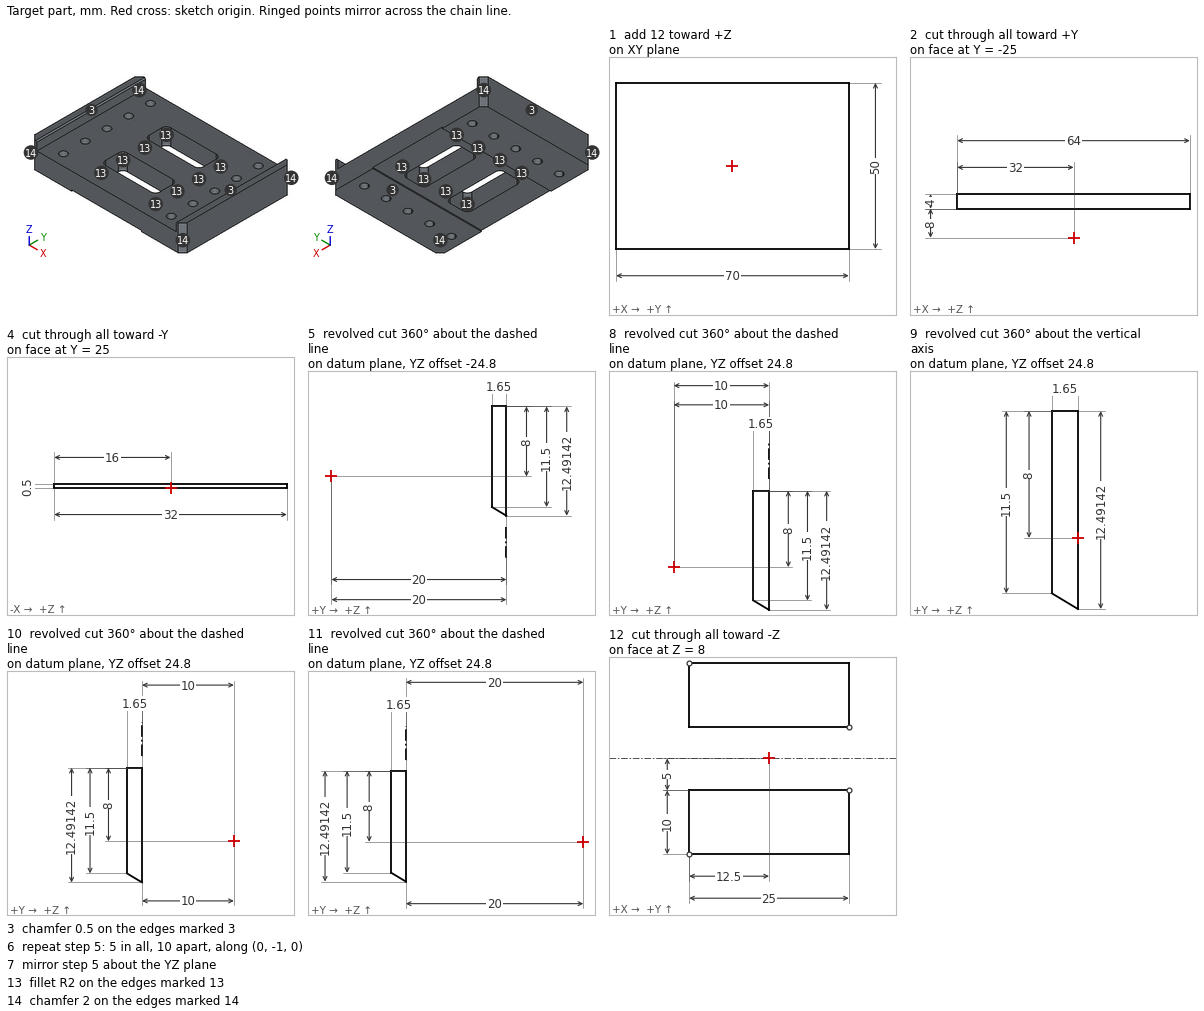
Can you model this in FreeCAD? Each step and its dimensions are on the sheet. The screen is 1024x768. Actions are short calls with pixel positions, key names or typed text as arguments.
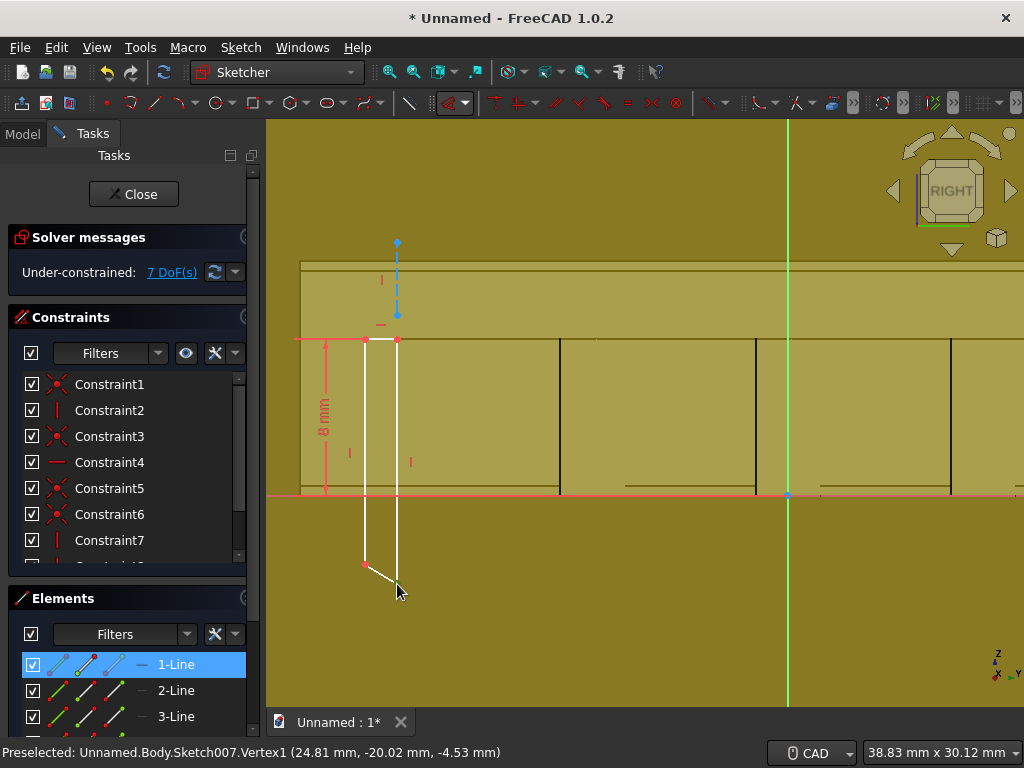
key(l)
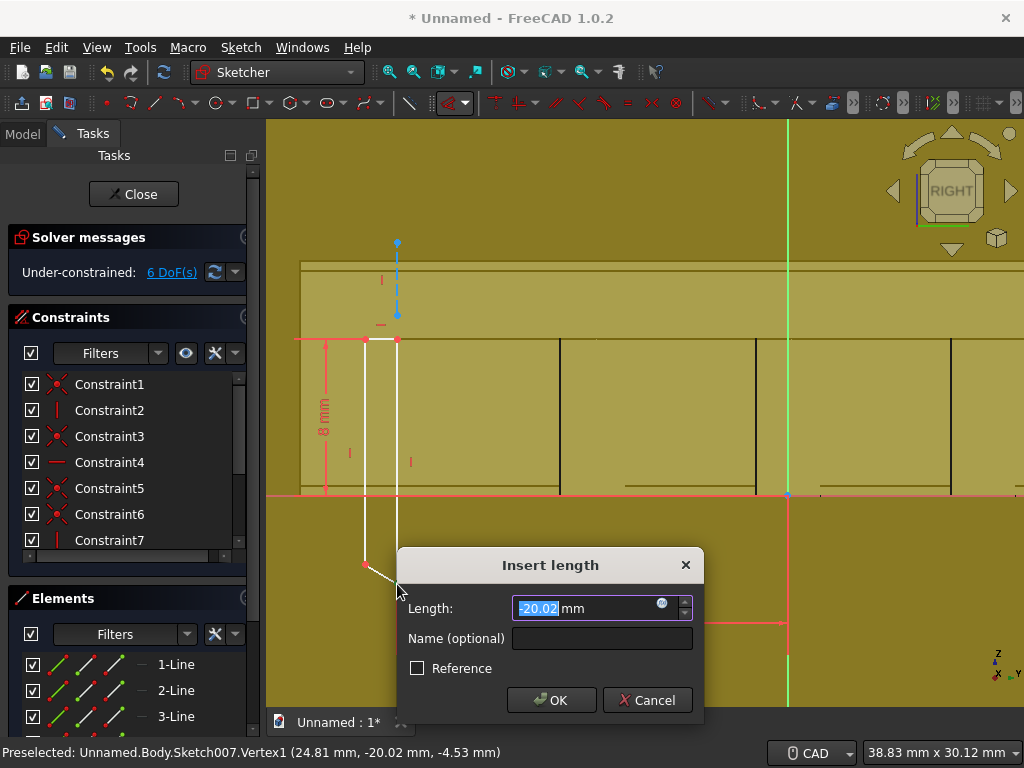
text(-20)
key(Return)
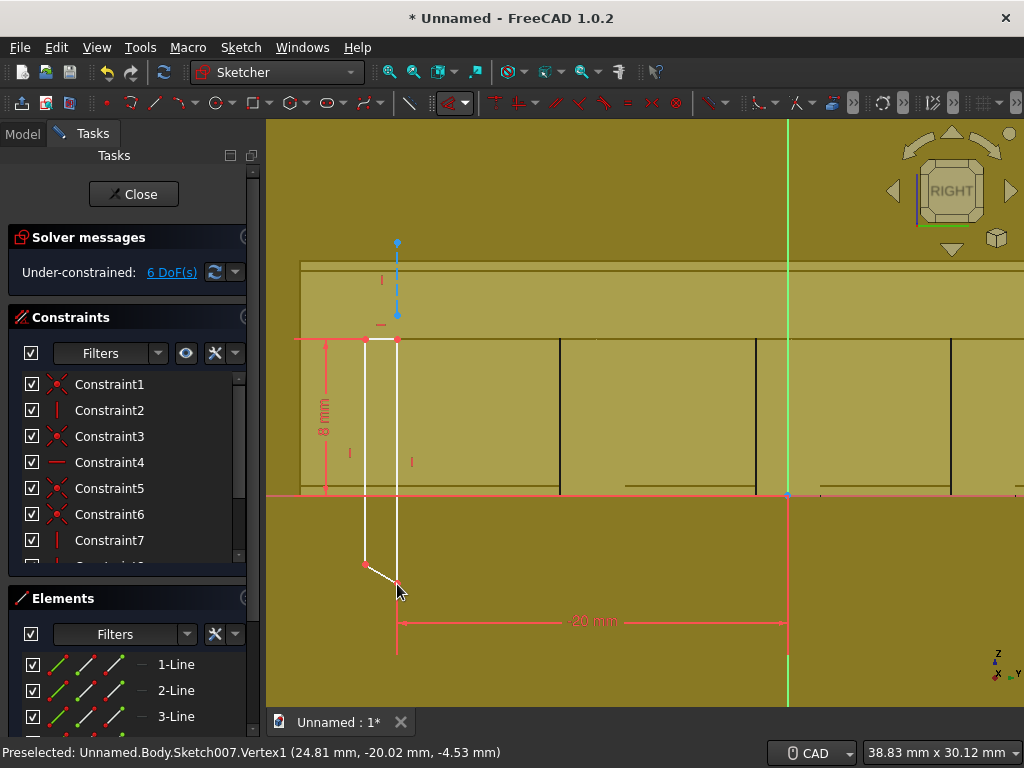
click(397, 316)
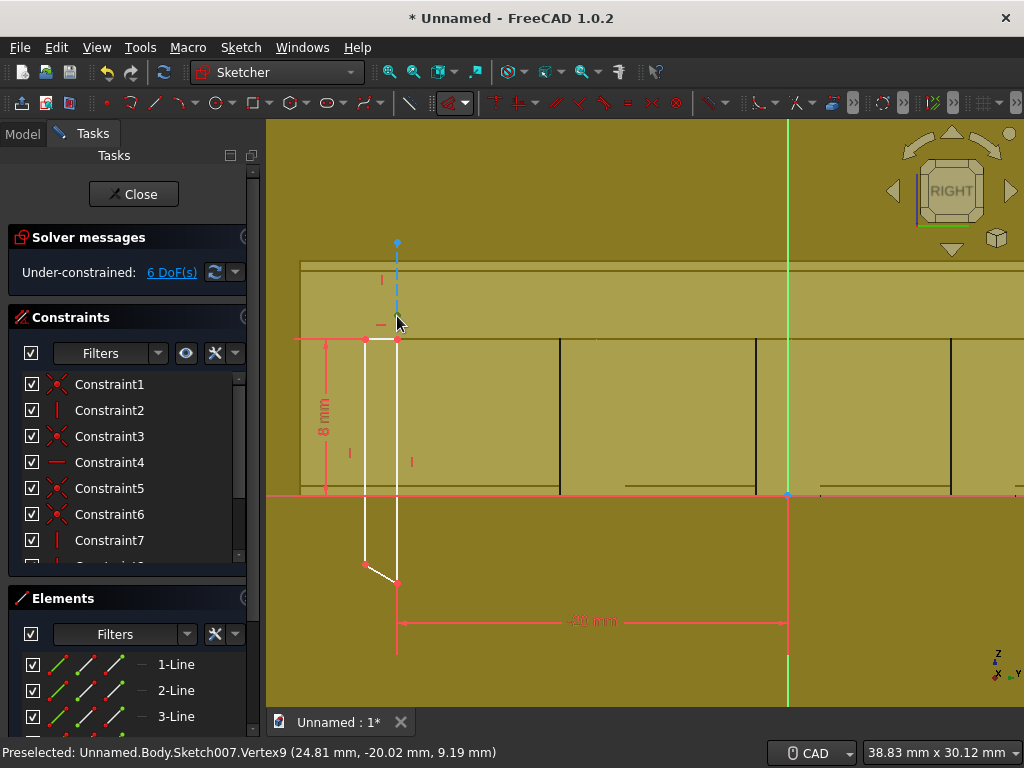
key(l)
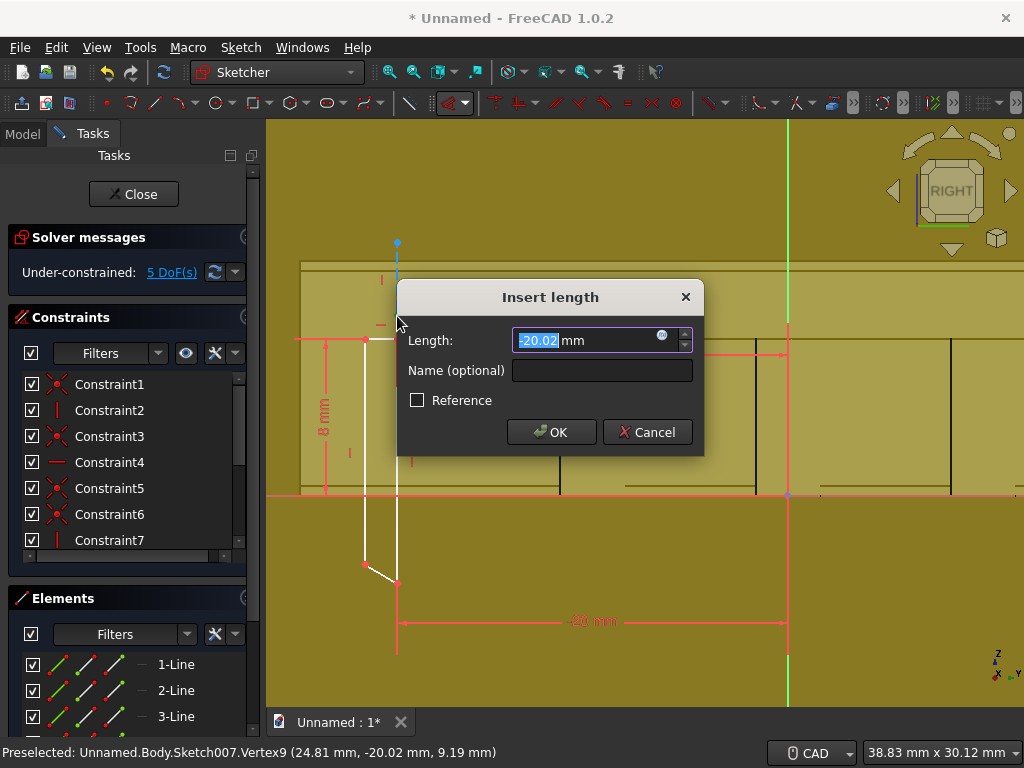
text(-20)
key(Return)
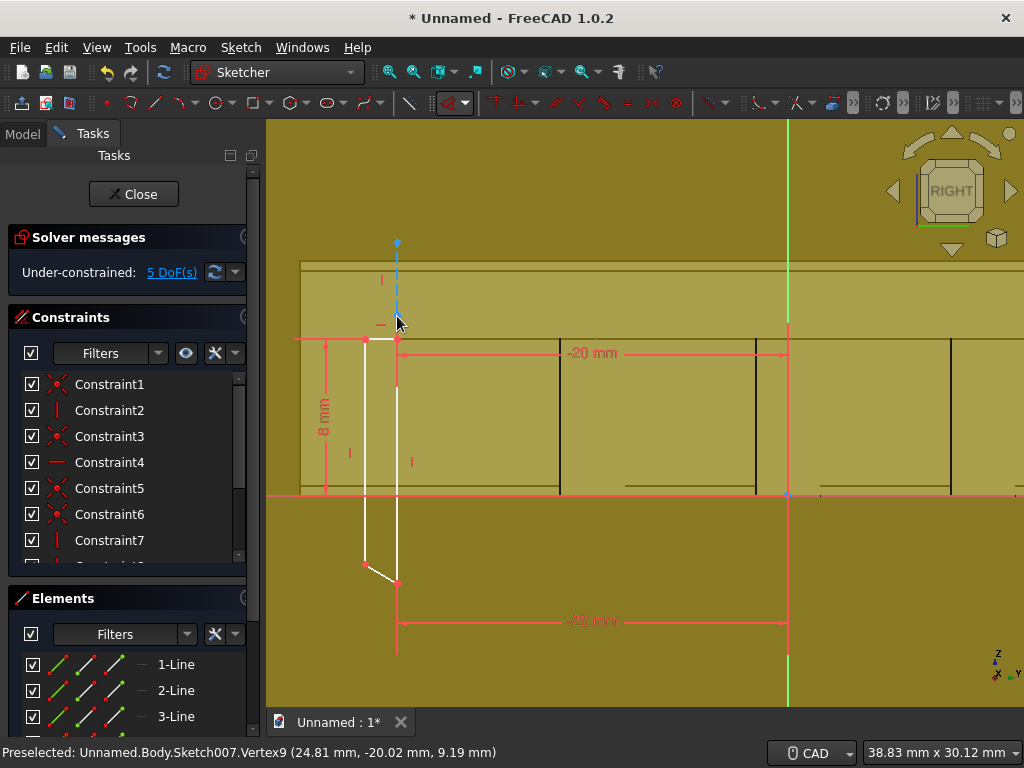
click(365, 497)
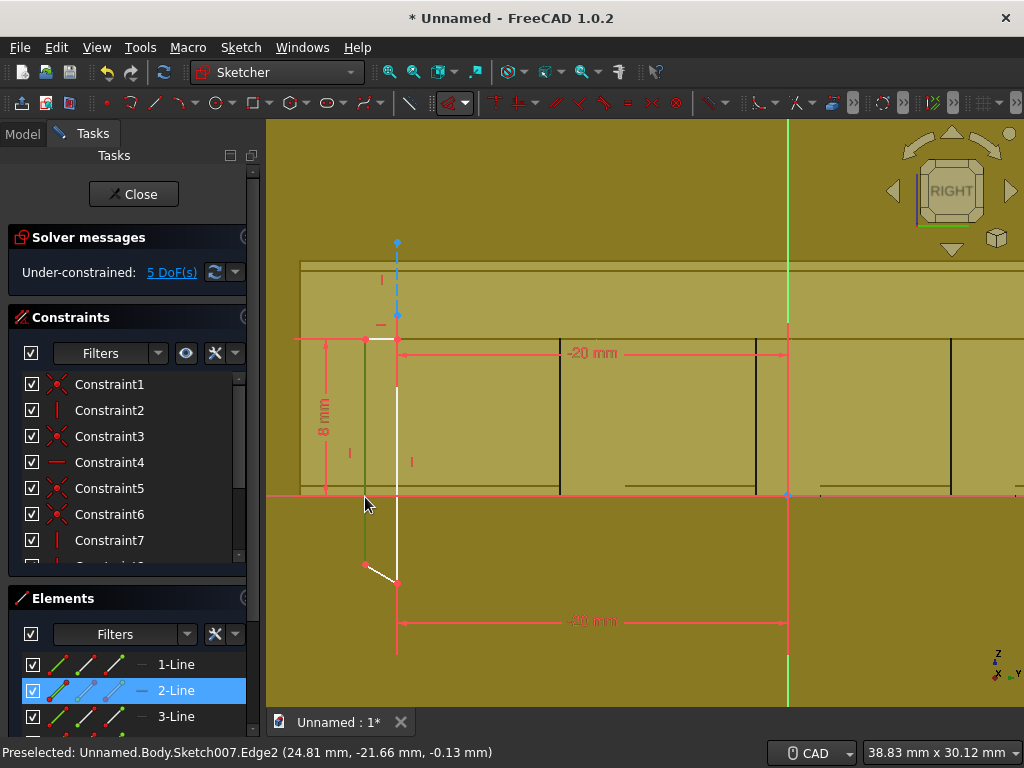
click(468, 104)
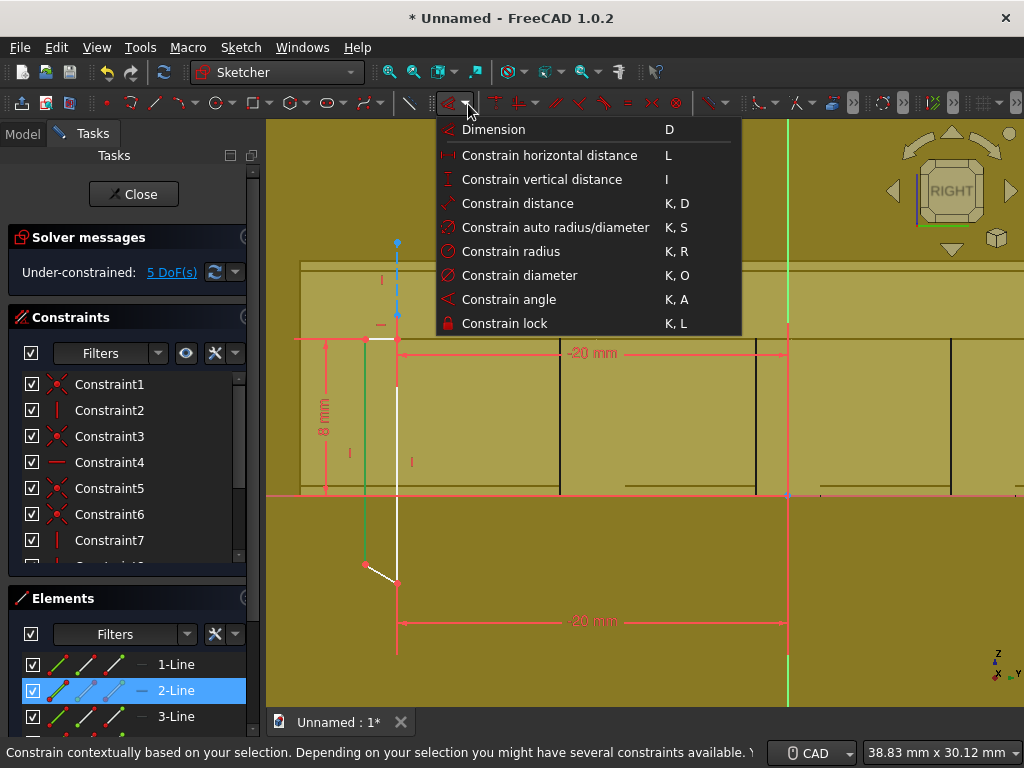
click(589, 179)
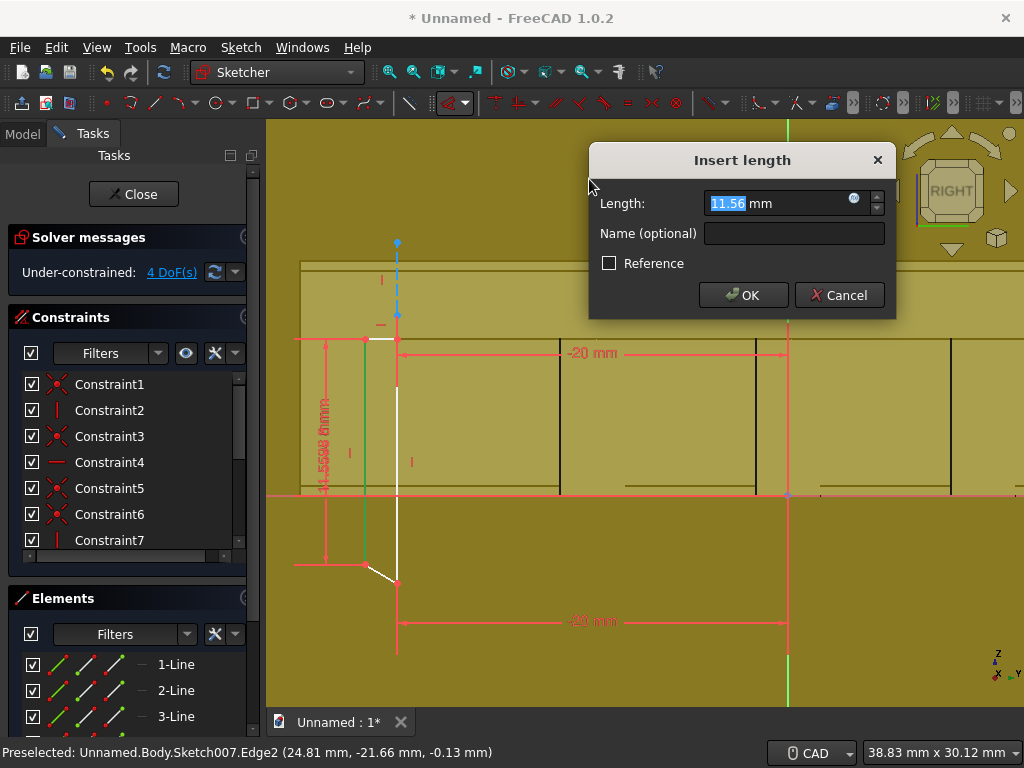
text(11.5)
key(Return)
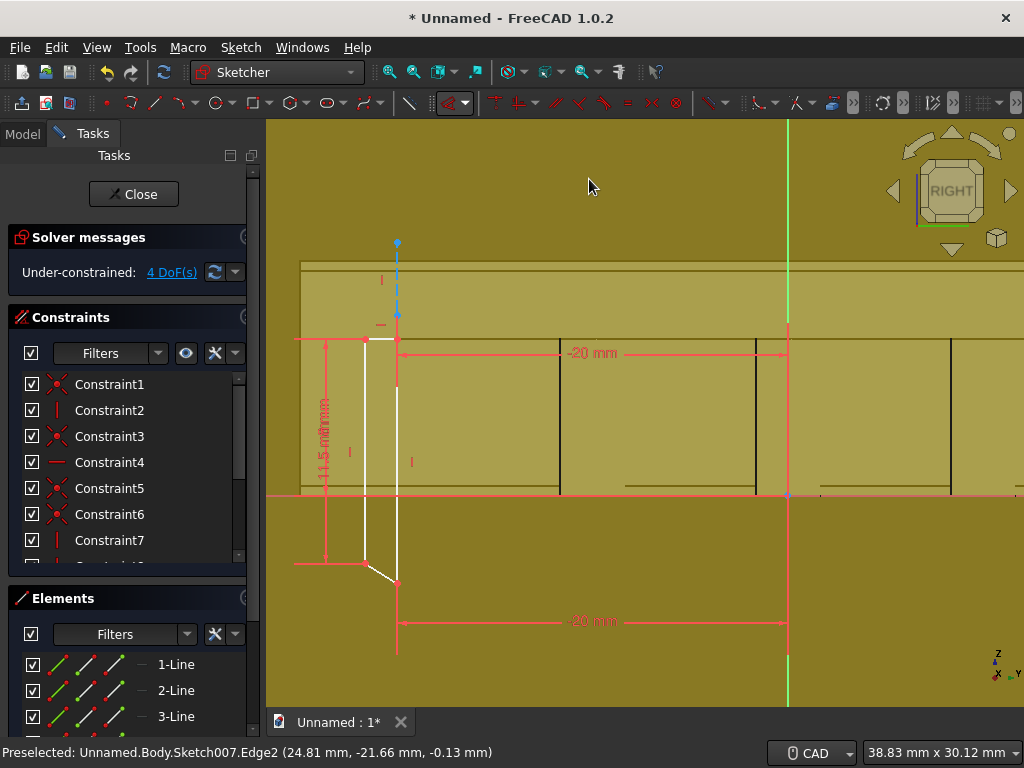
scroll(375, 339, up, 2)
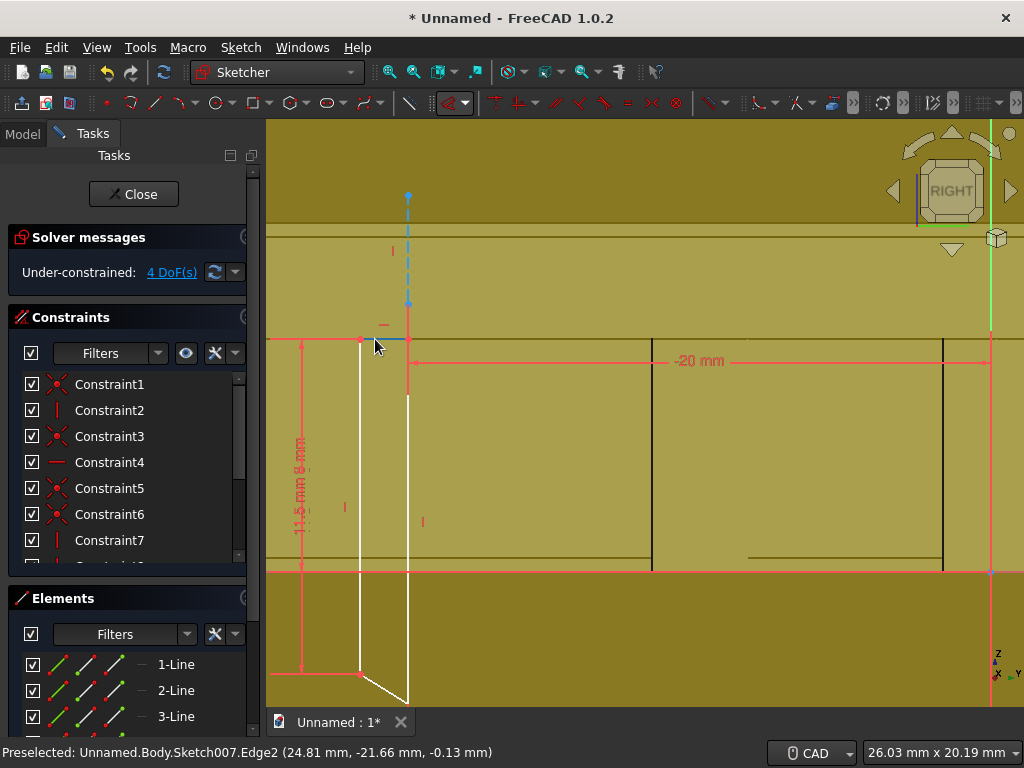
click(375, 339)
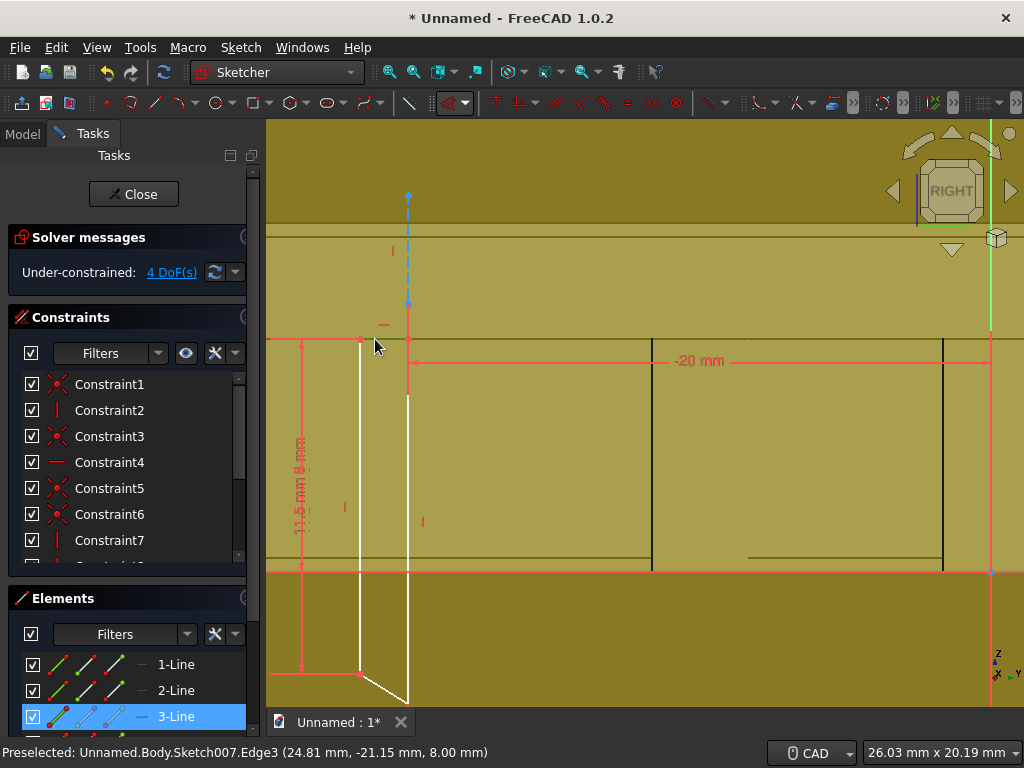
key(l)